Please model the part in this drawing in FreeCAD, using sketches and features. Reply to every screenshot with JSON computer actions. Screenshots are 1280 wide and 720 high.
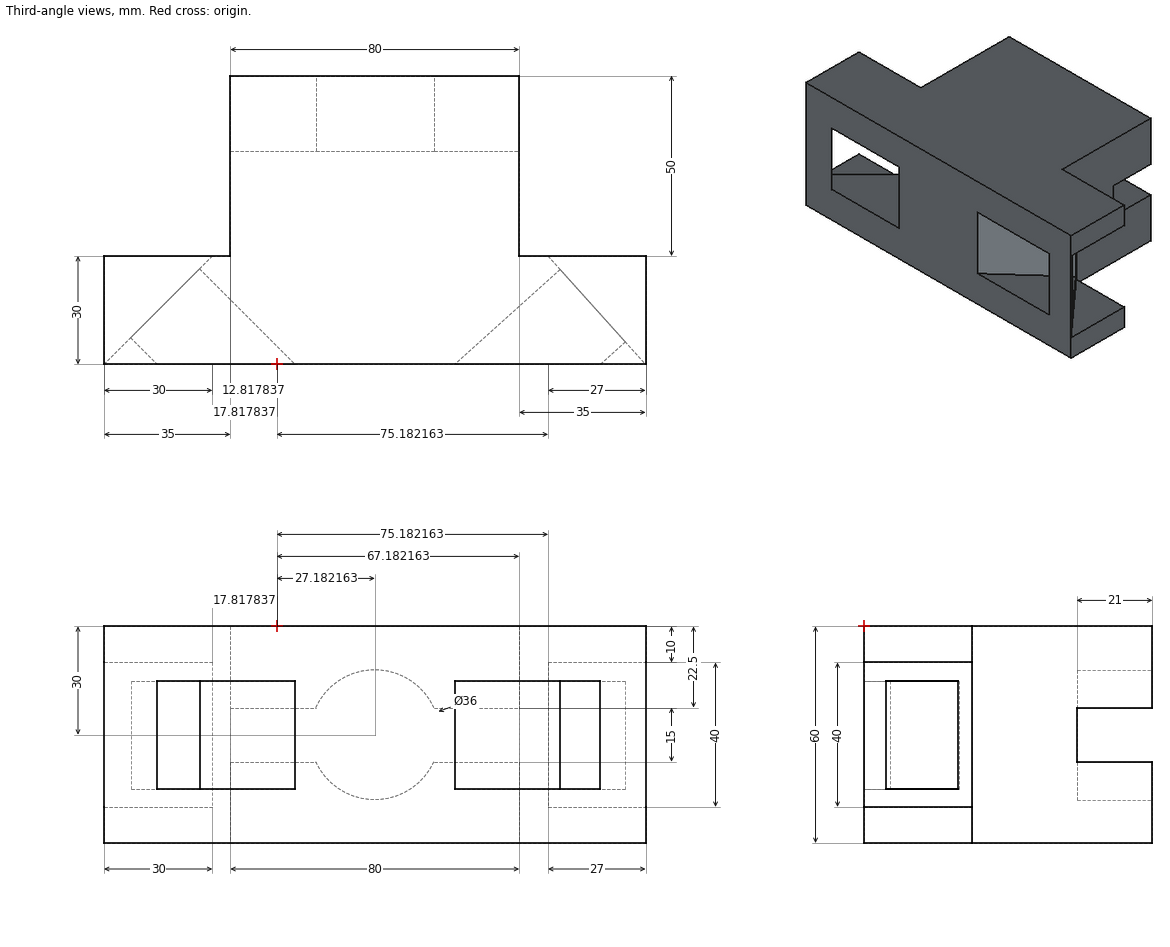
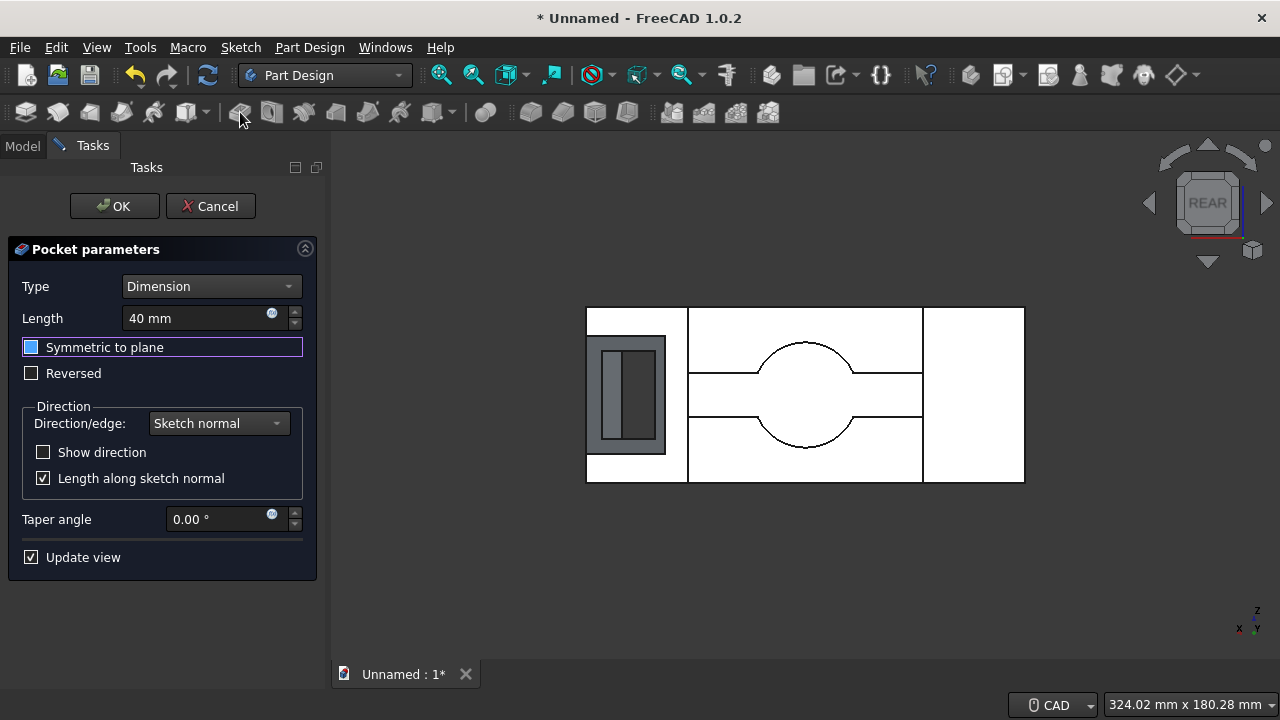
{"action": "left_click", "coordinate": [115, 206]}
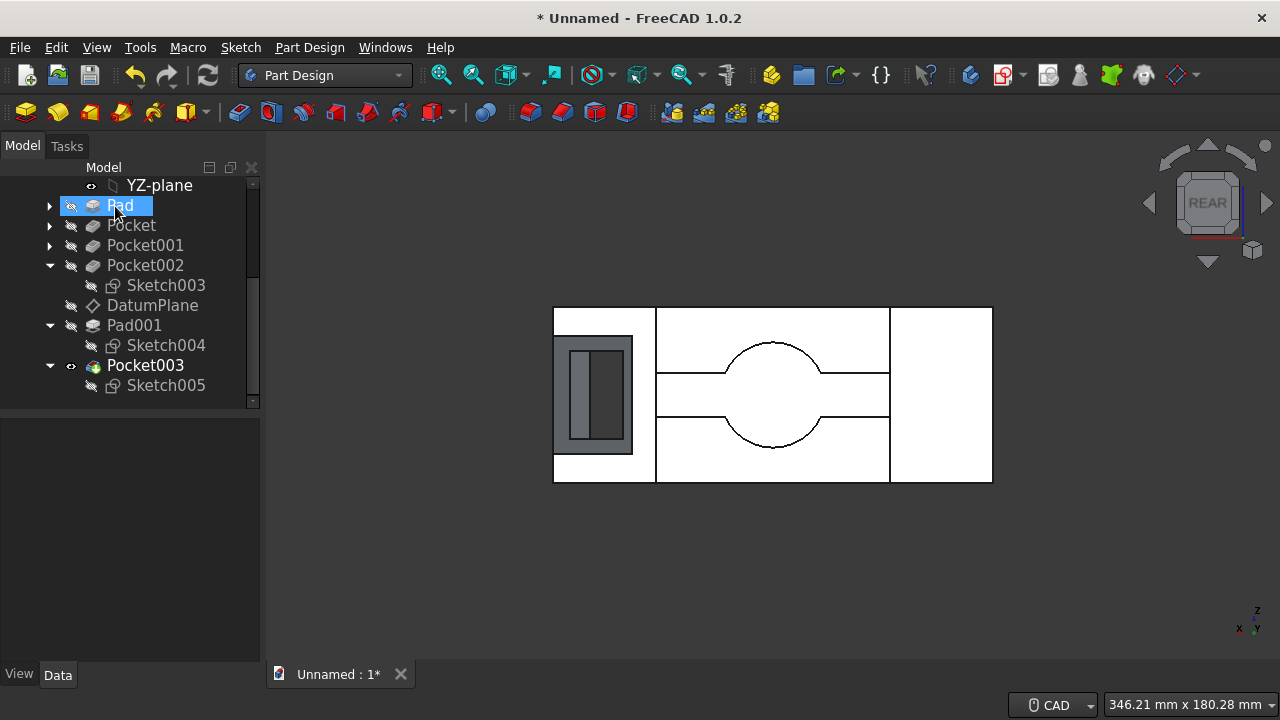
{"action": "left_click", "coordinate": [442, 76]}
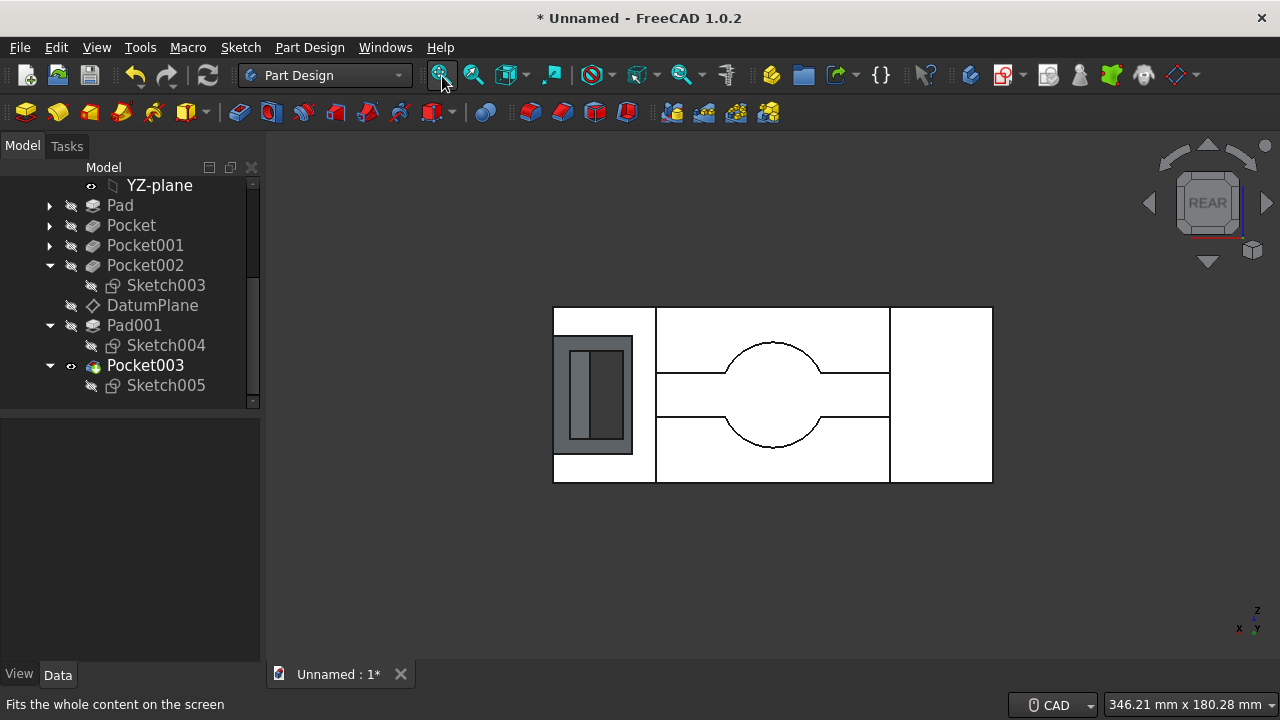
{"action": "left_click", "coordinate": [941, 369]}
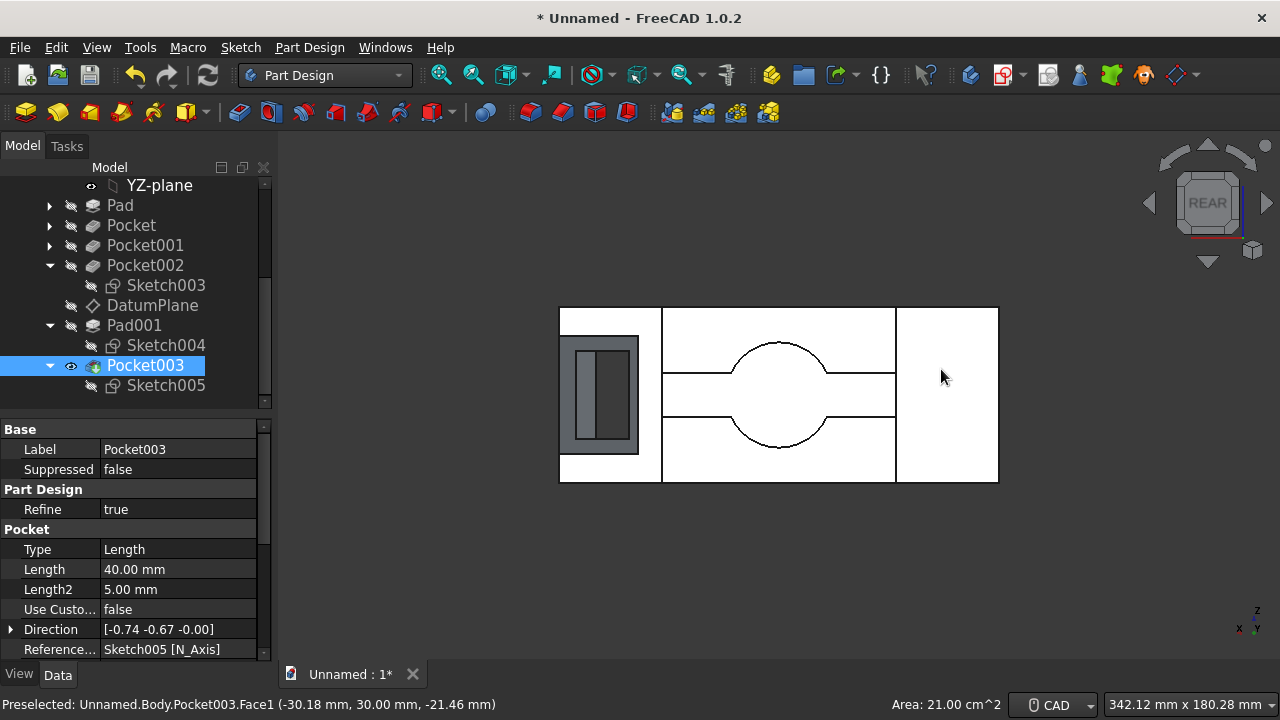
{"action": "left_click", "coordinate": [1004, 76]}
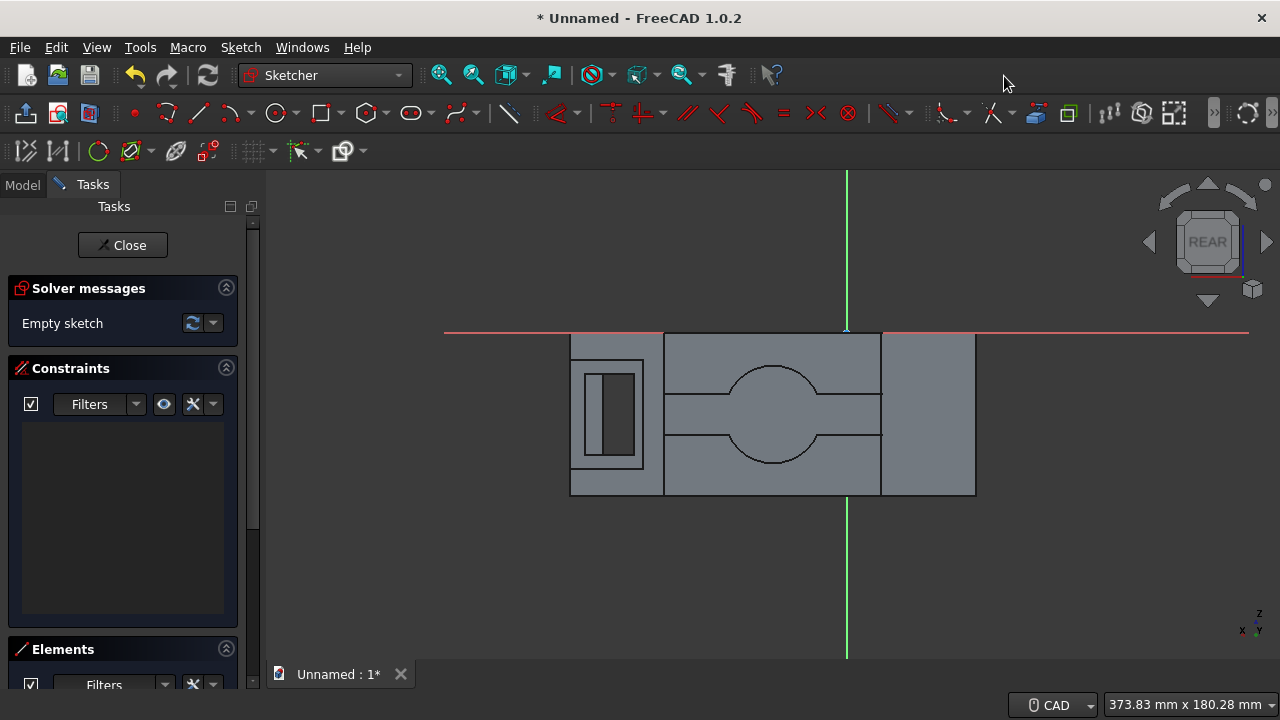
{"action": "left_click", "coordinate": [90, 114]}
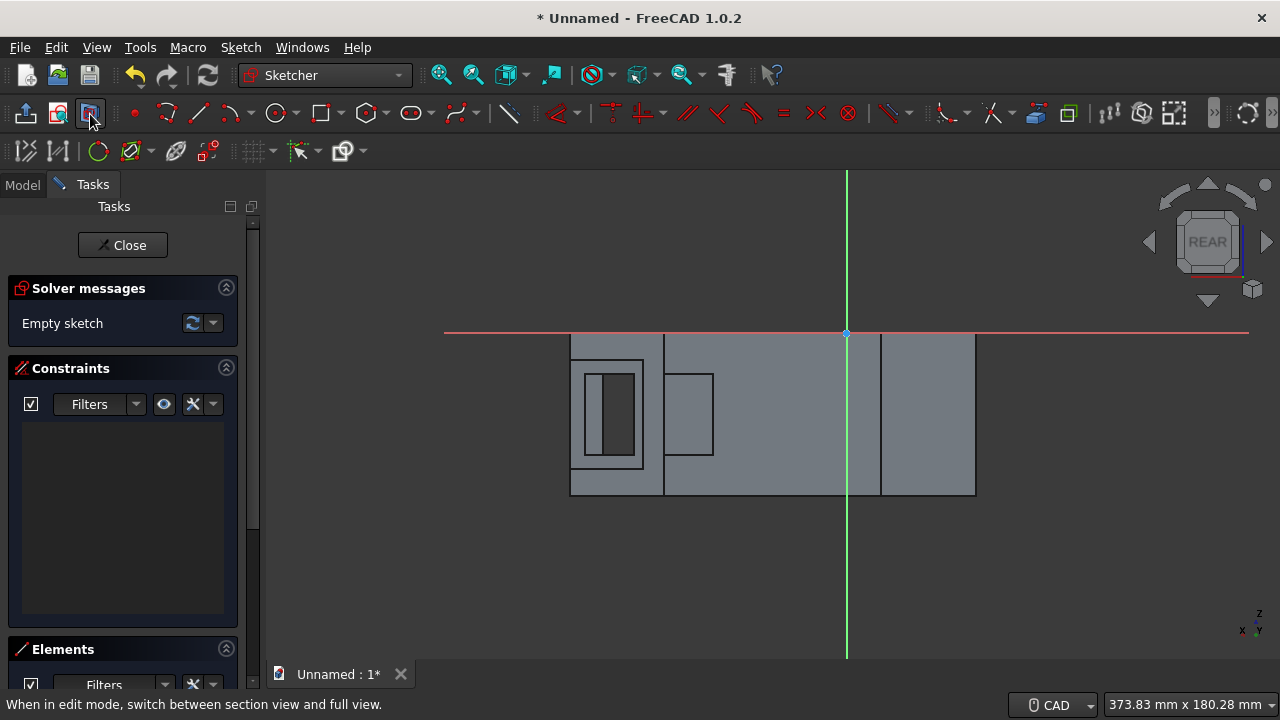
{"action": "scroll", "coordinate": [1081, 390], "scroll_direction": "up", "scroll_amount": 4}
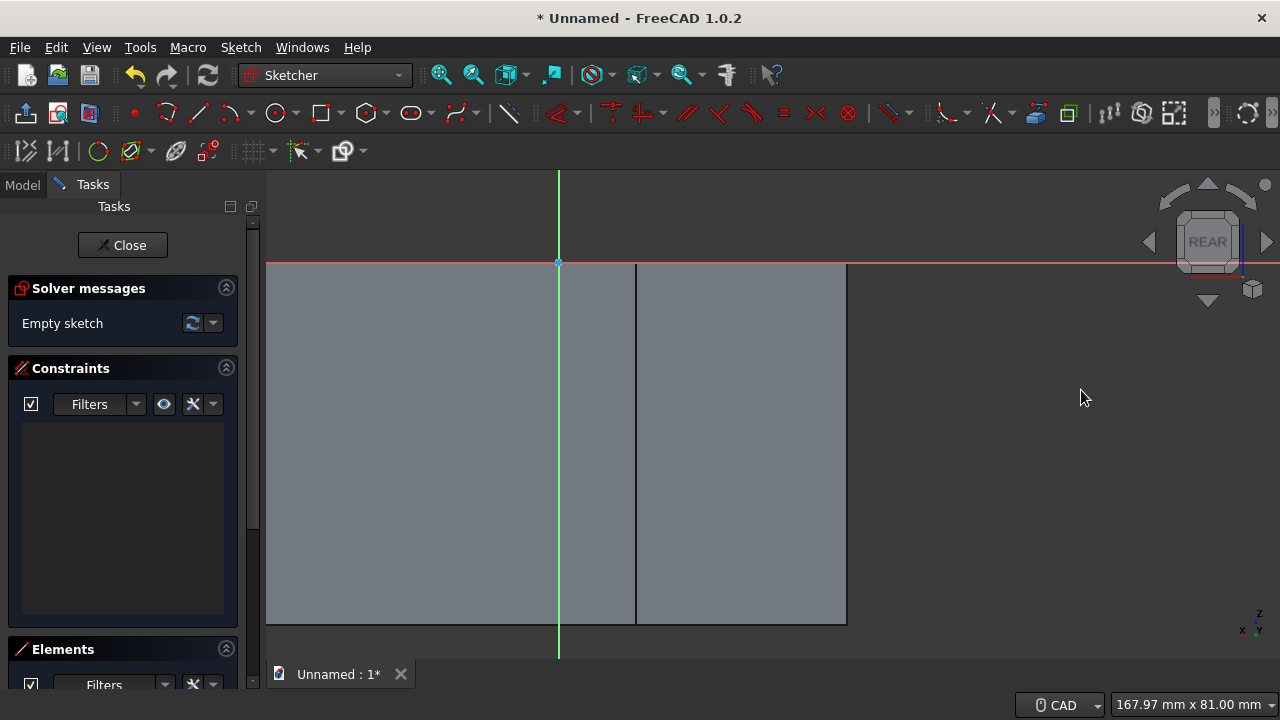
{"action": "left_click", "coordinate": [322, 114]}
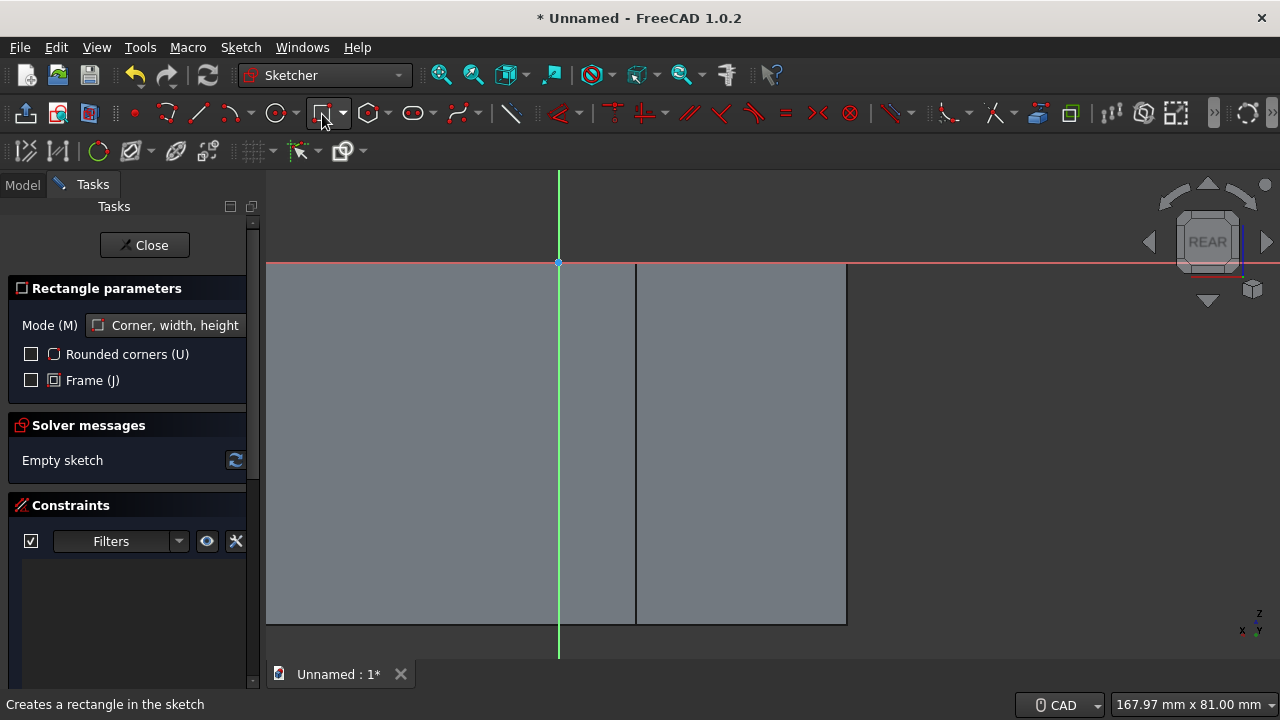
{"action": "left_click", "coordinate": [666, 323]}
{"action": "left_click", "coordinate": [847, 565]}
{"action": "key", "text": "Escape"}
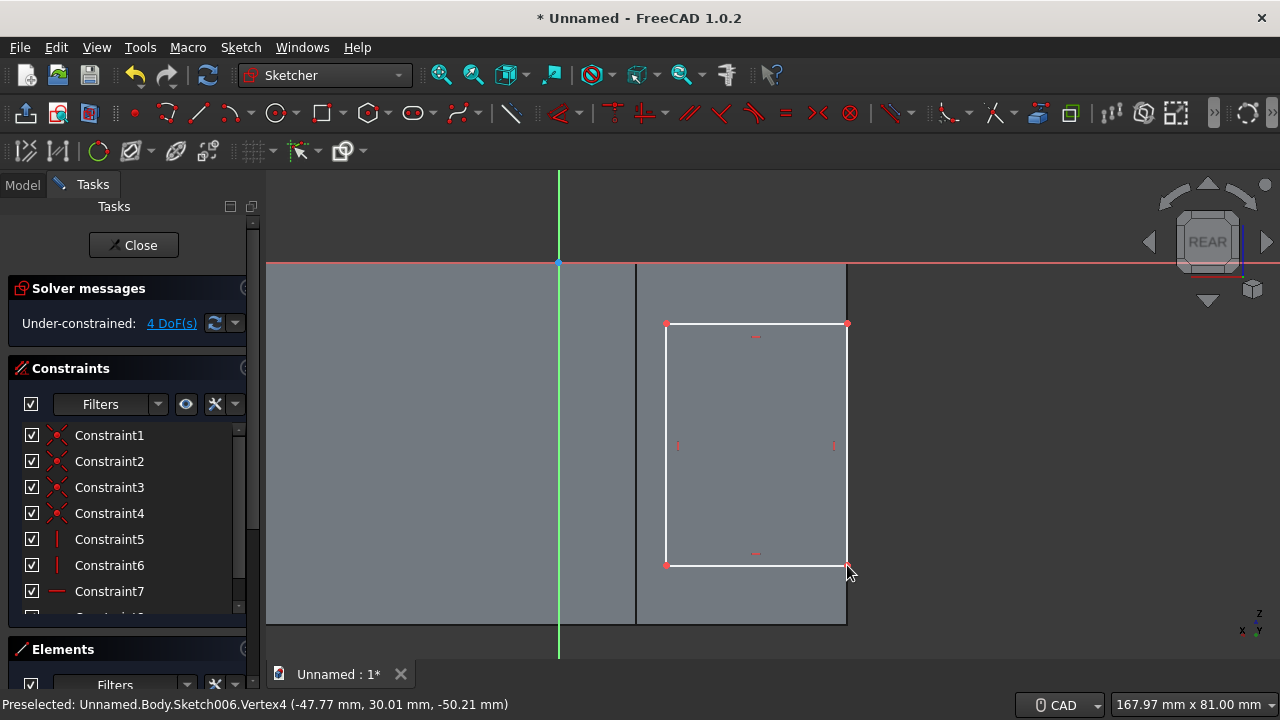
{"action": "left_click", "coordinate": [558, 114]}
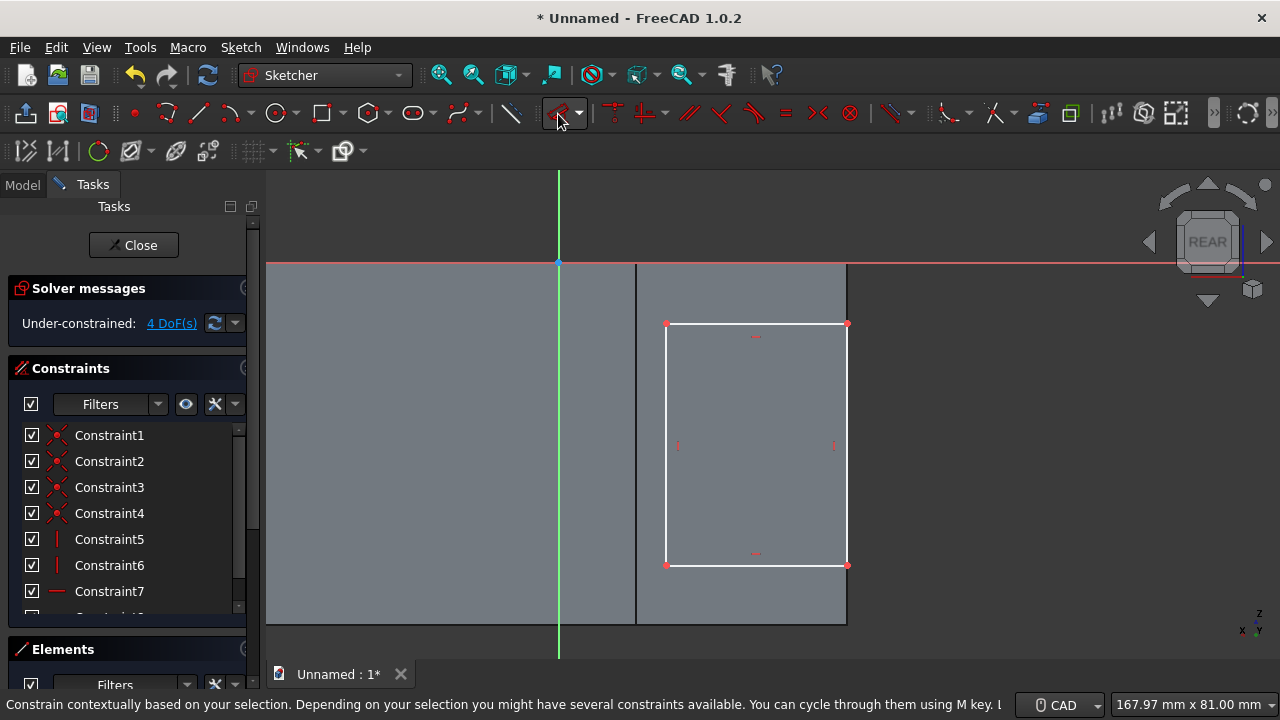
{"action": "left_click", "coordinate": [666, 397]}
{"action": "left_click", "coordinate": [632, 445]}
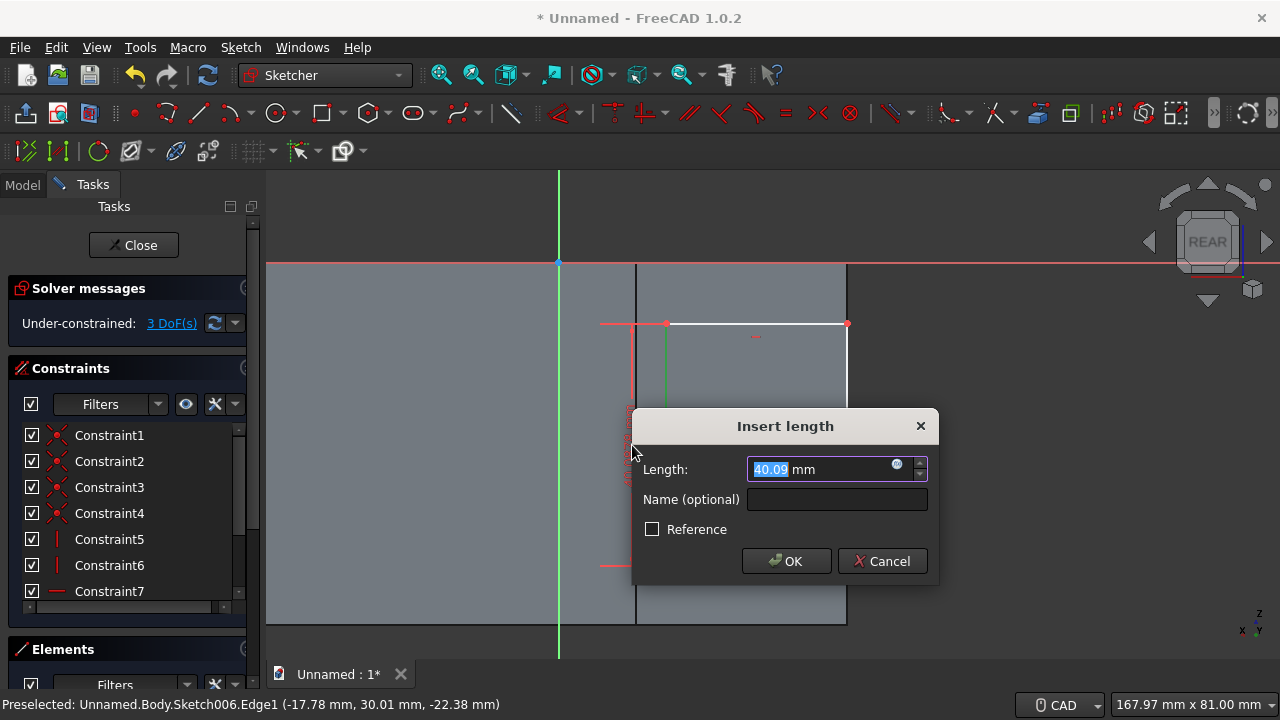
{"action": "type", "text": "40"}
{"action": "key", "text": "Return"}